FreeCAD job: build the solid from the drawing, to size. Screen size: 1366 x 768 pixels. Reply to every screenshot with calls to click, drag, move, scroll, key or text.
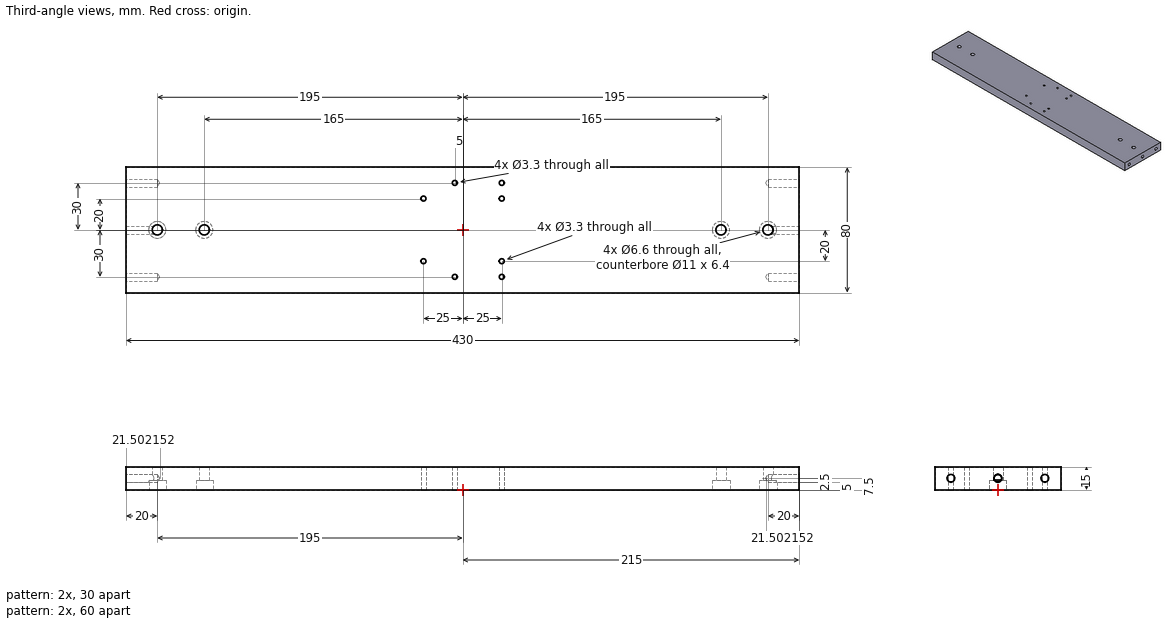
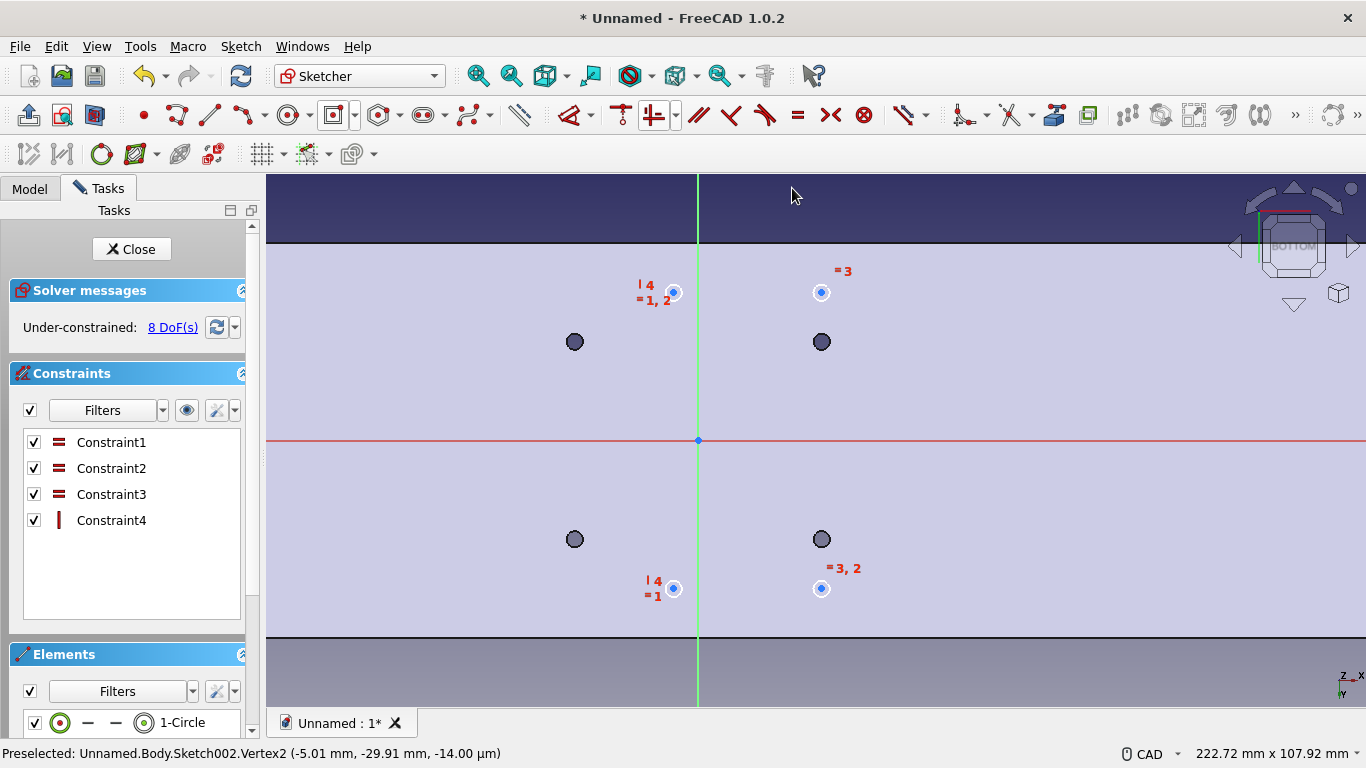
click(674, 589)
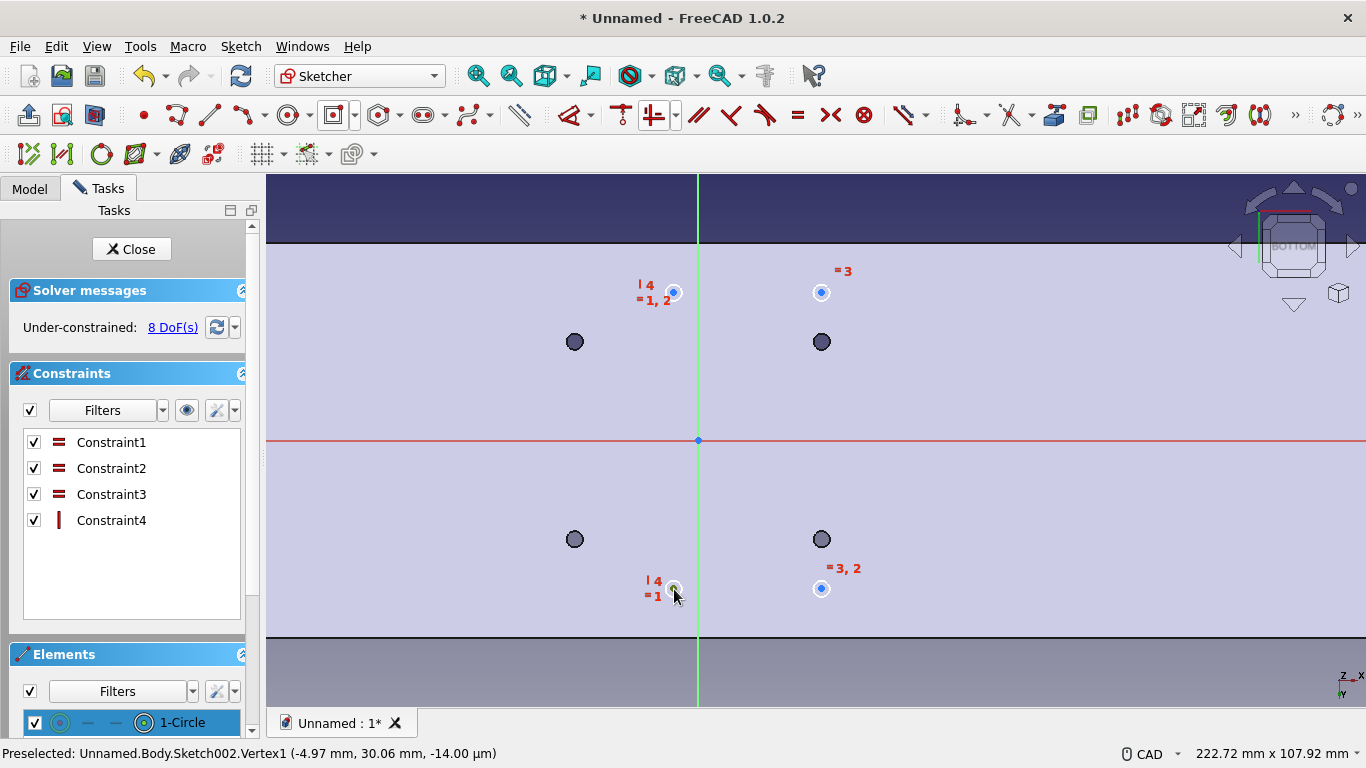
click(822, 589)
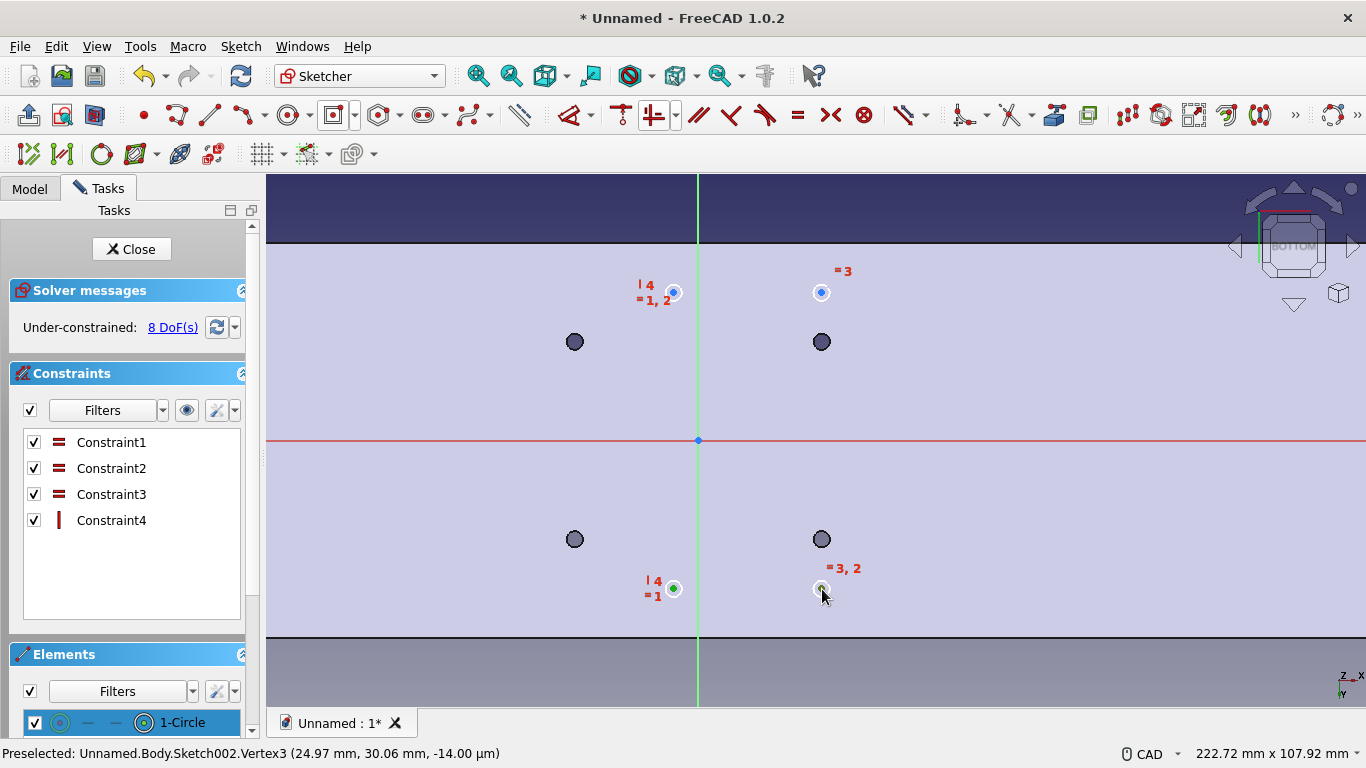
click(676, 116)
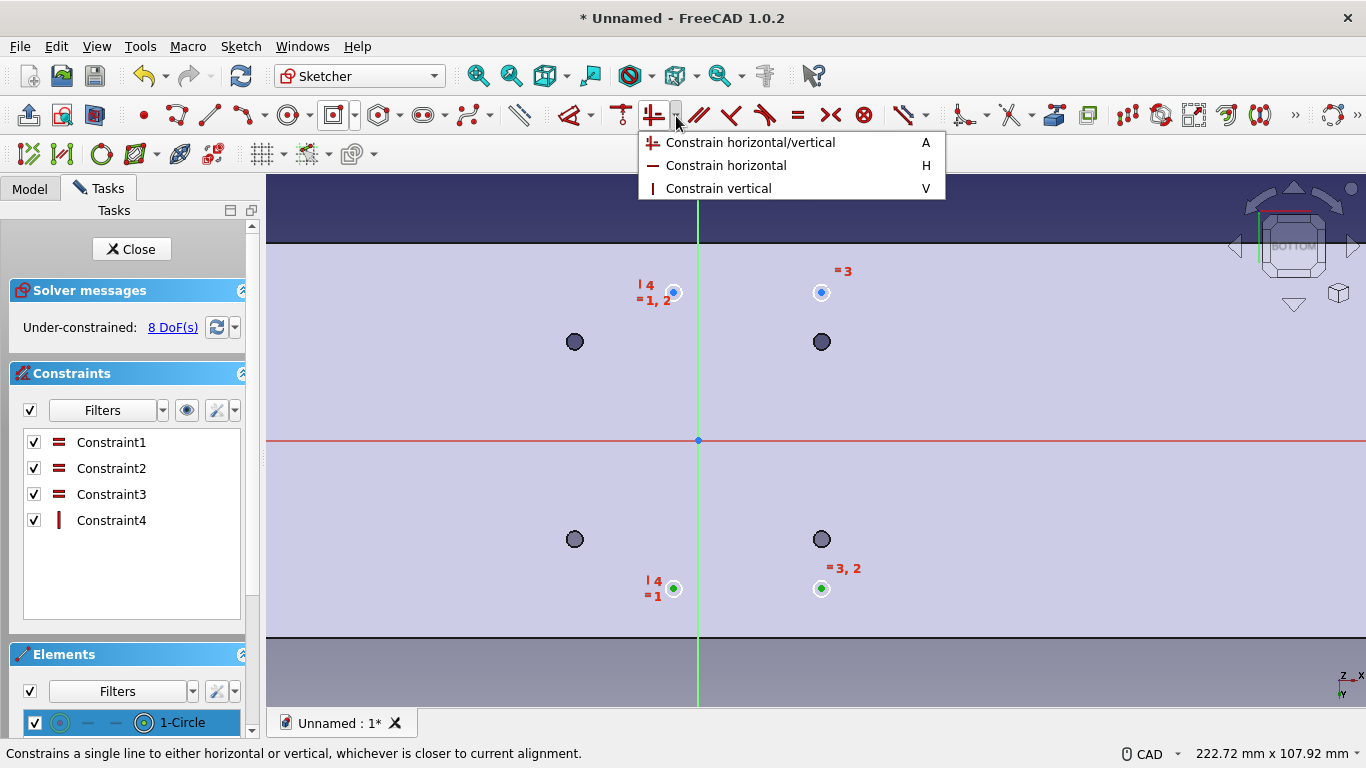
click(792, 166)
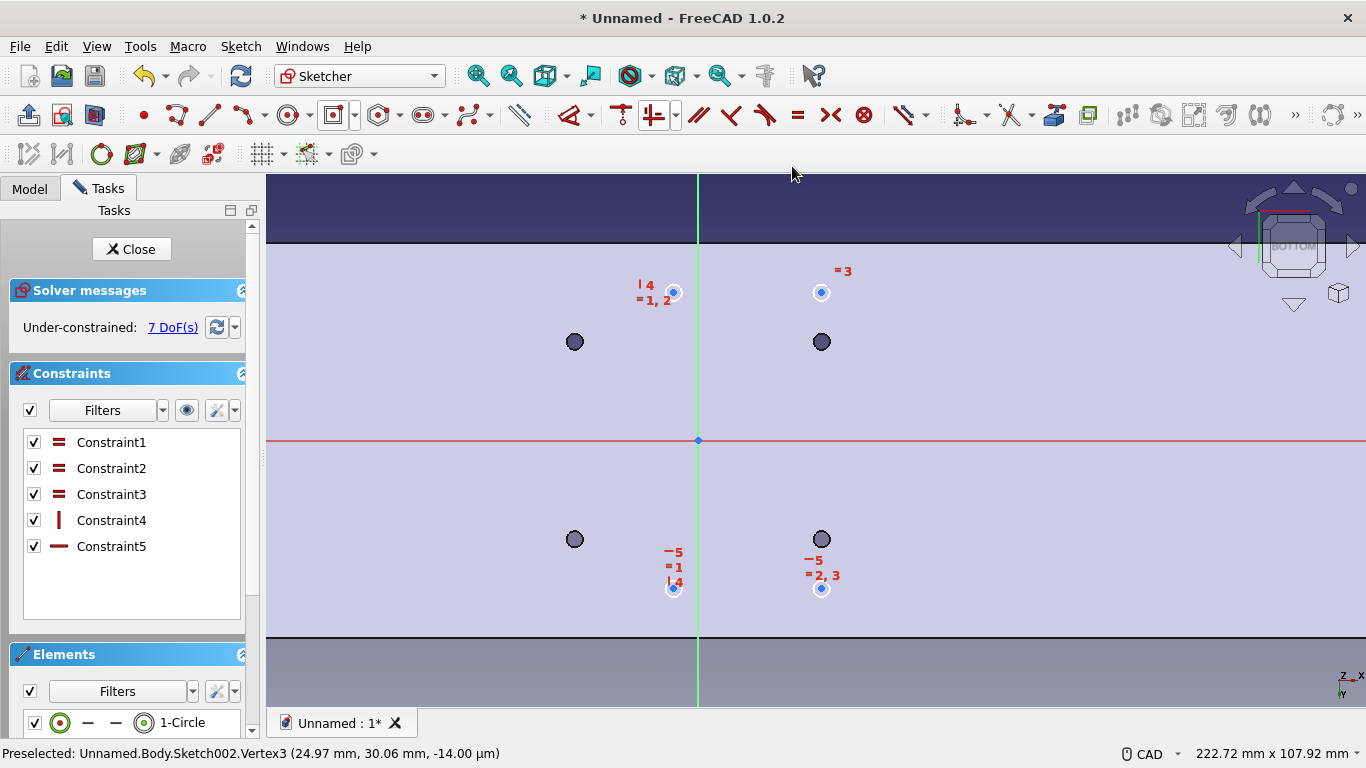
click(822, 589)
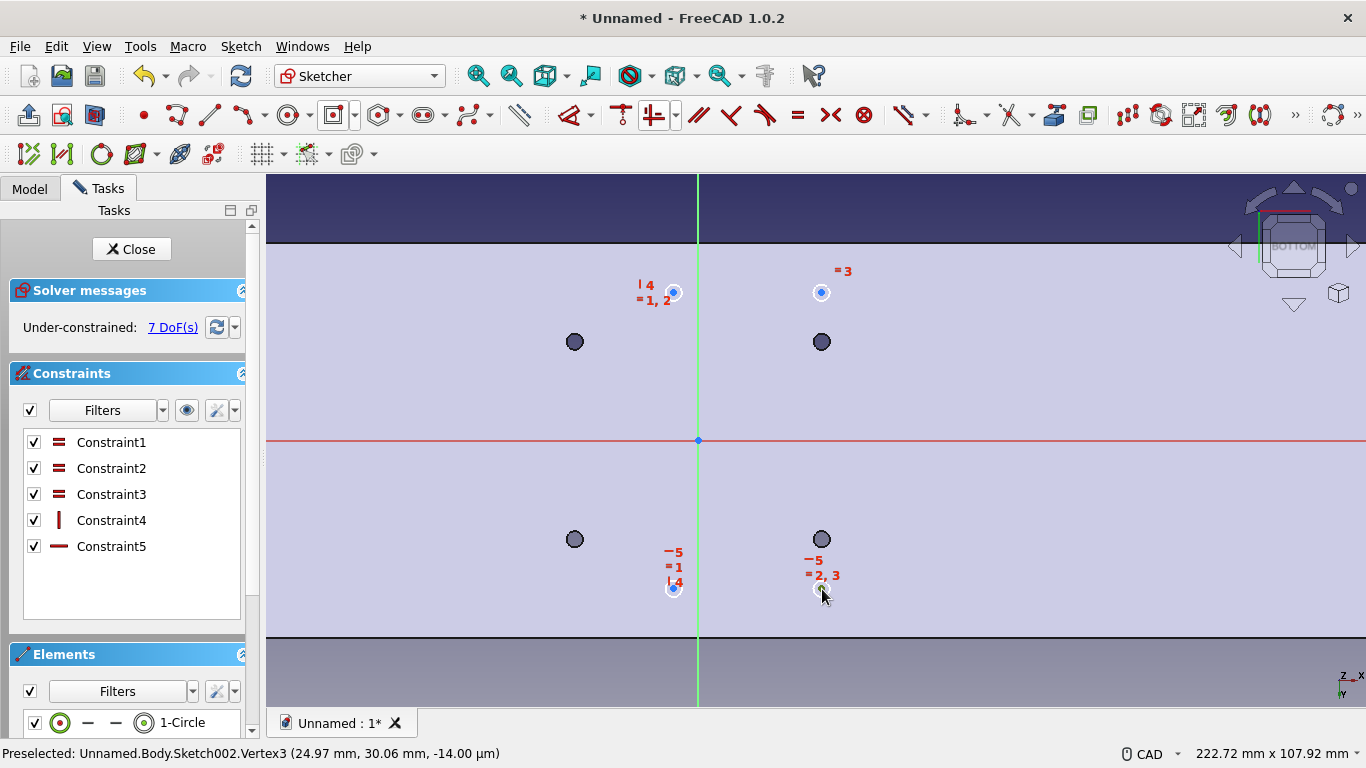
click(822, 293)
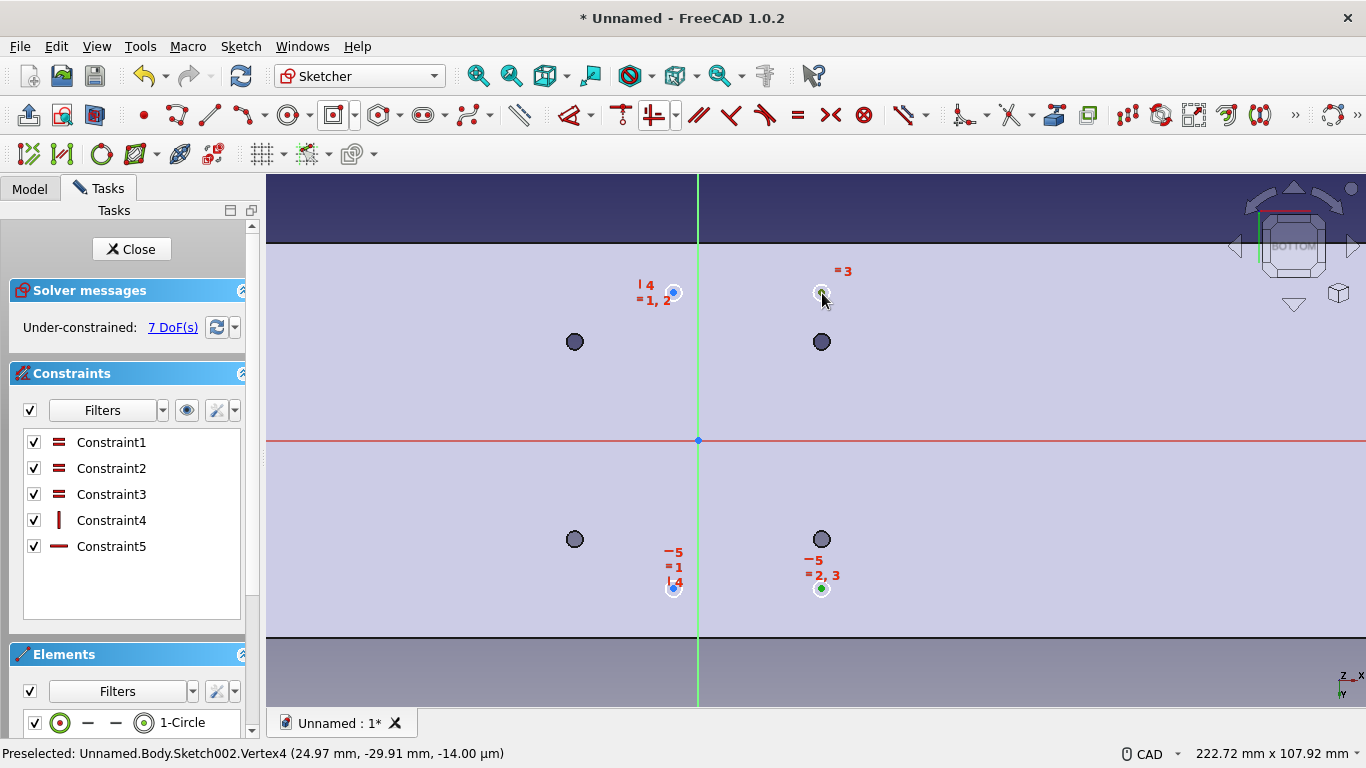
key(v)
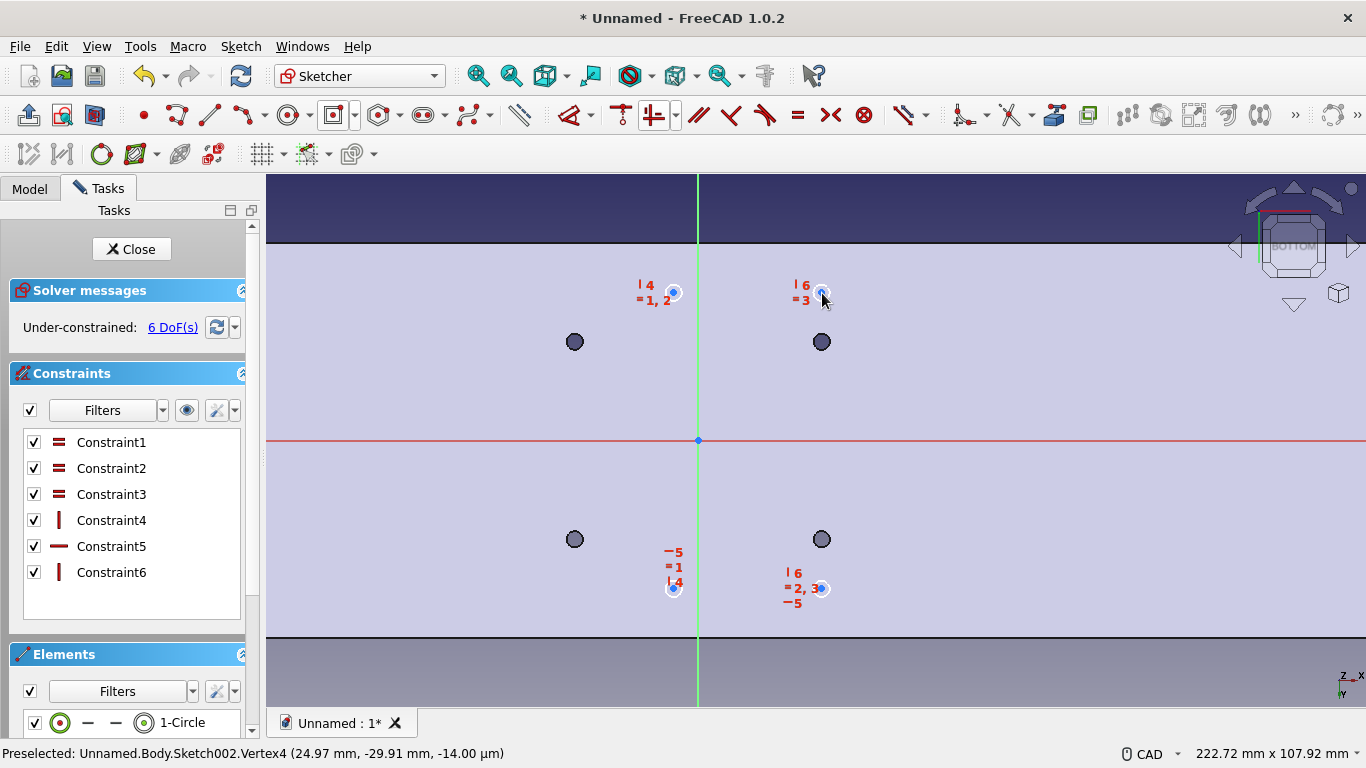
click(674, 293)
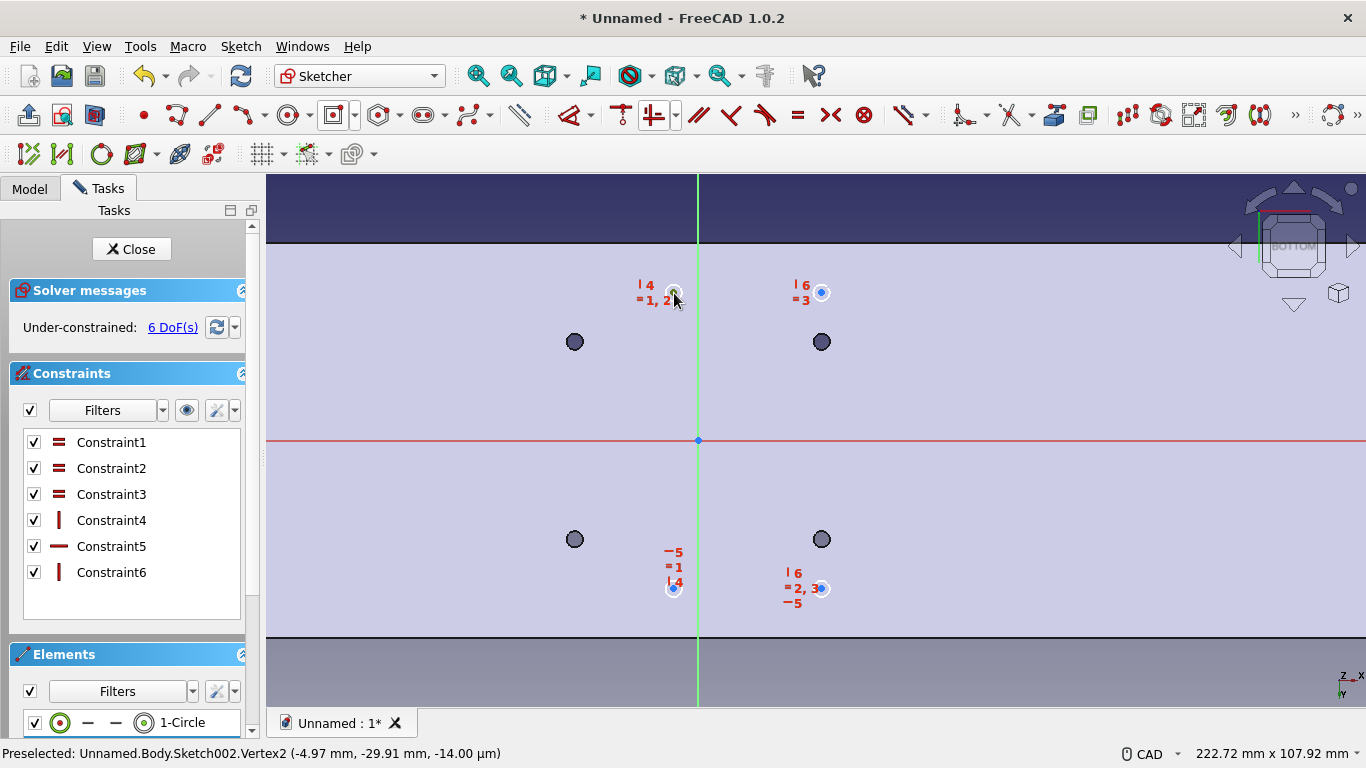
click(822, 293)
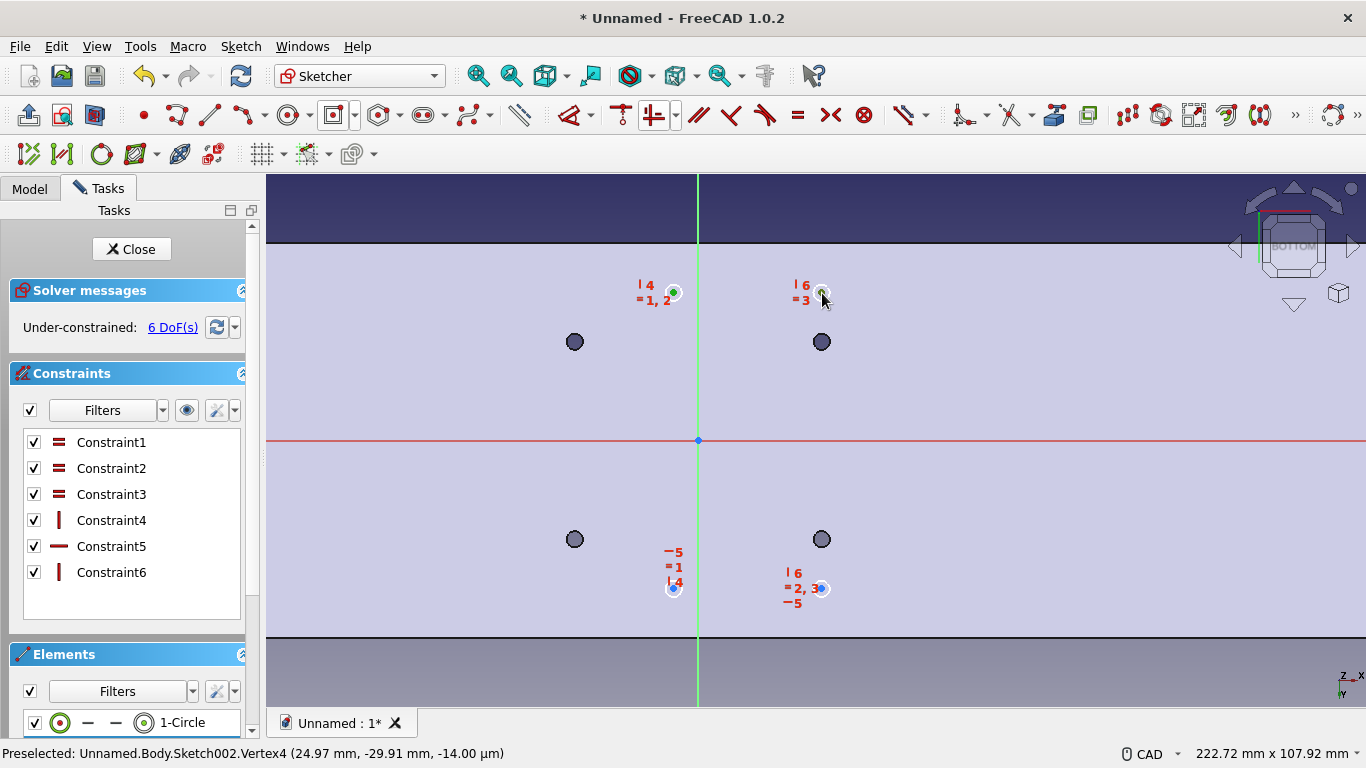
key(h)